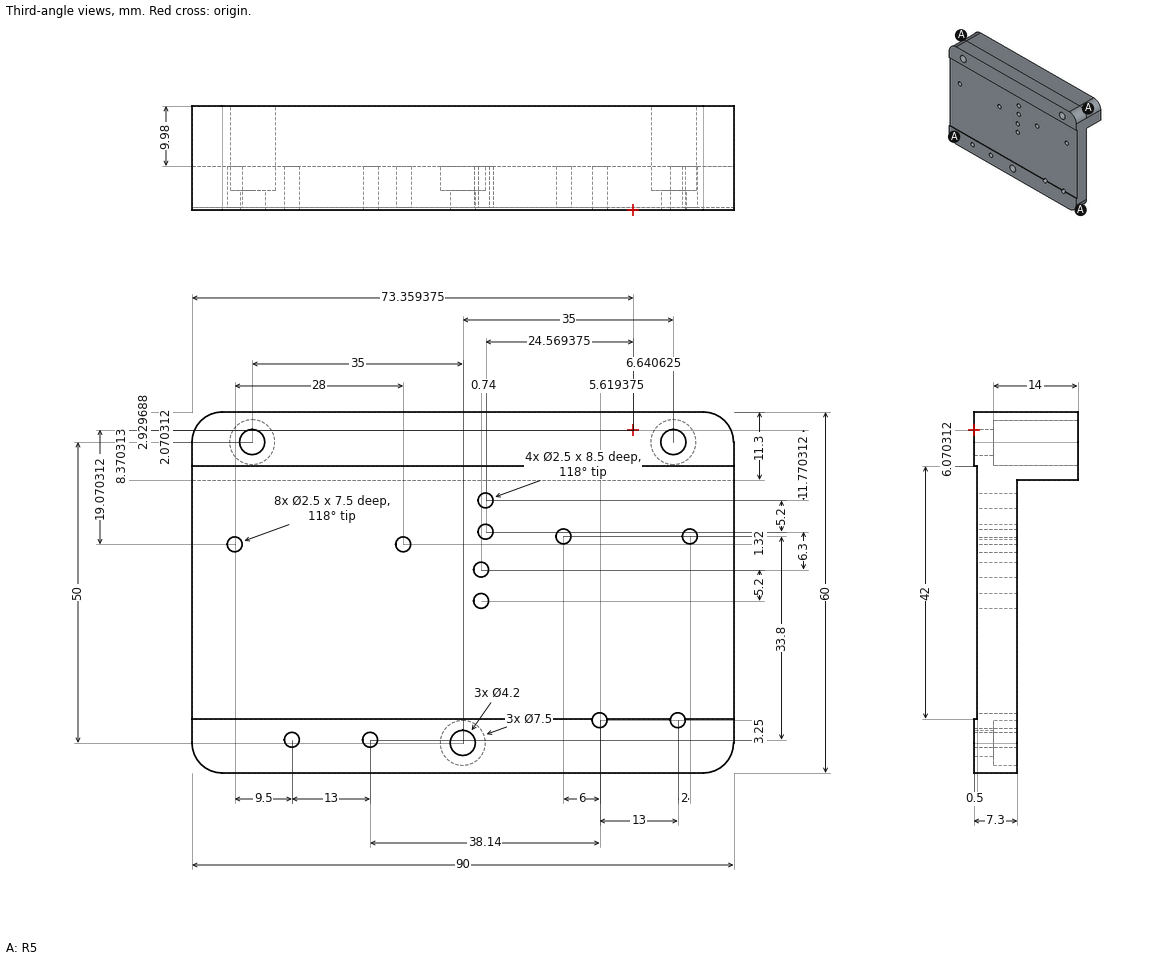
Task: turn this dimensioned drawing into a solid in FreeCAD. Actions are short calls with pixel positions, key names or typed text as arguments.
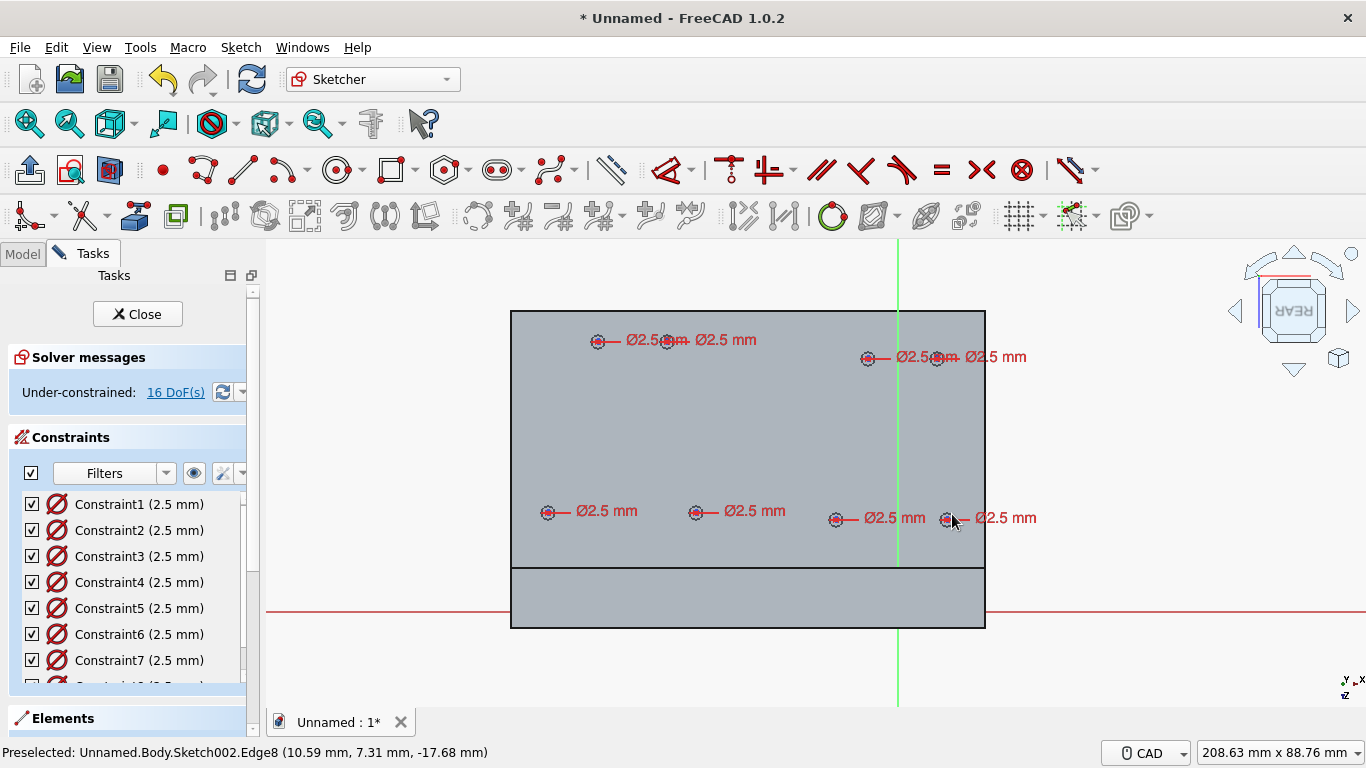
click(666, 170)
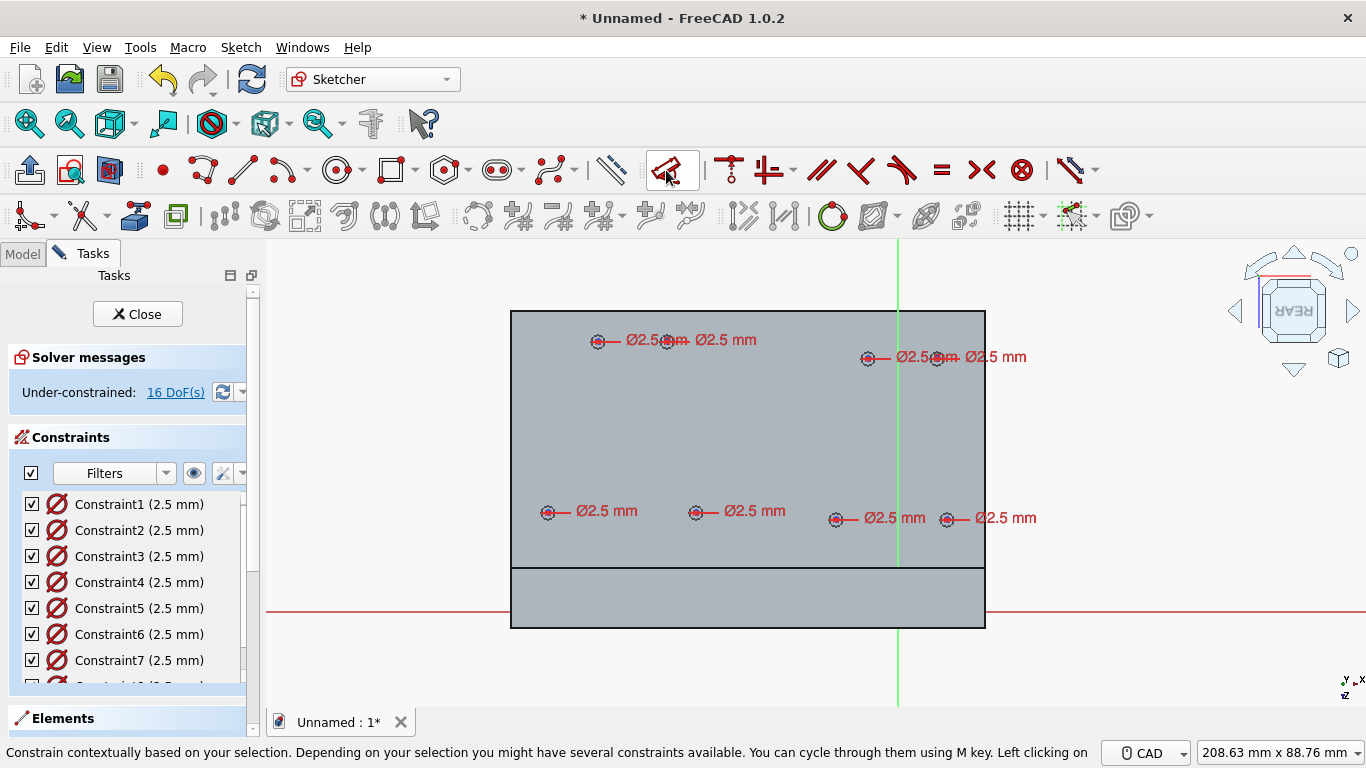
scroll(868, 359, up, 2)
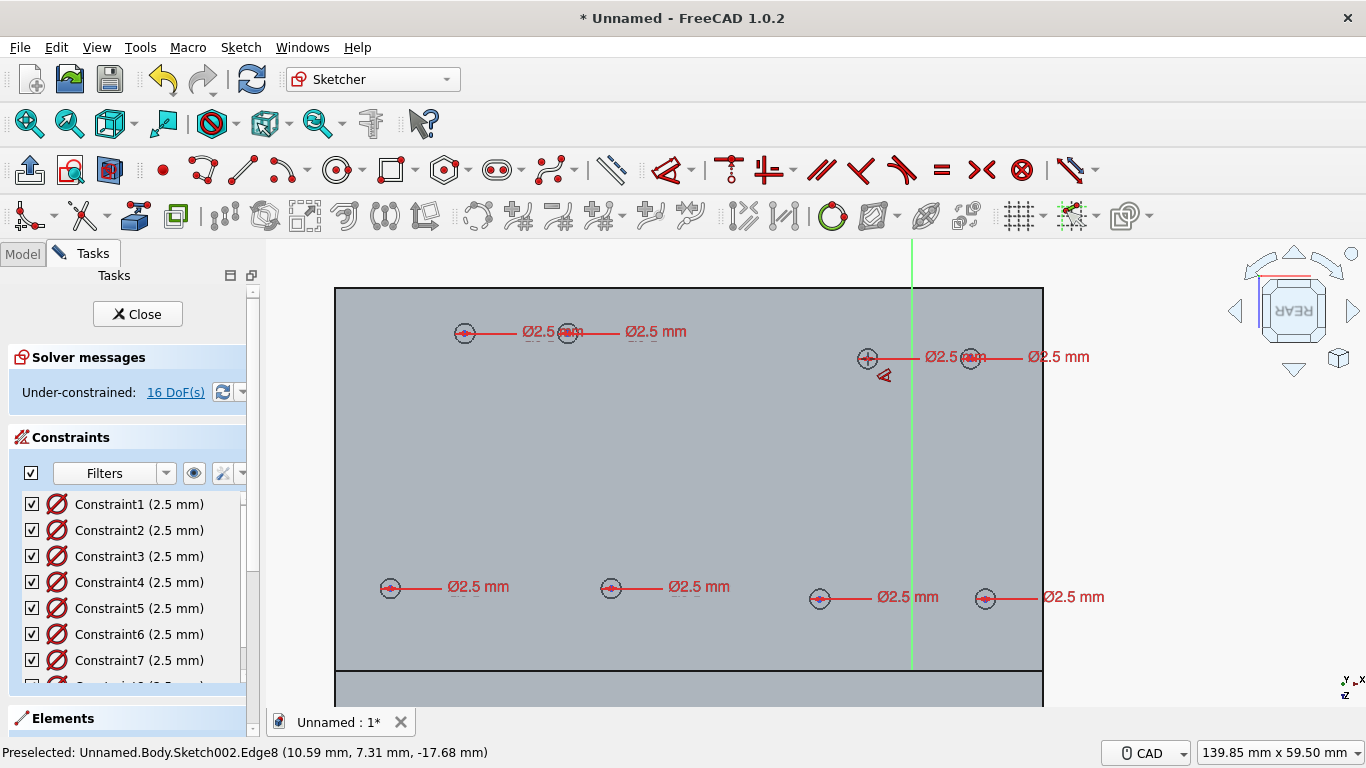
click(868, 359)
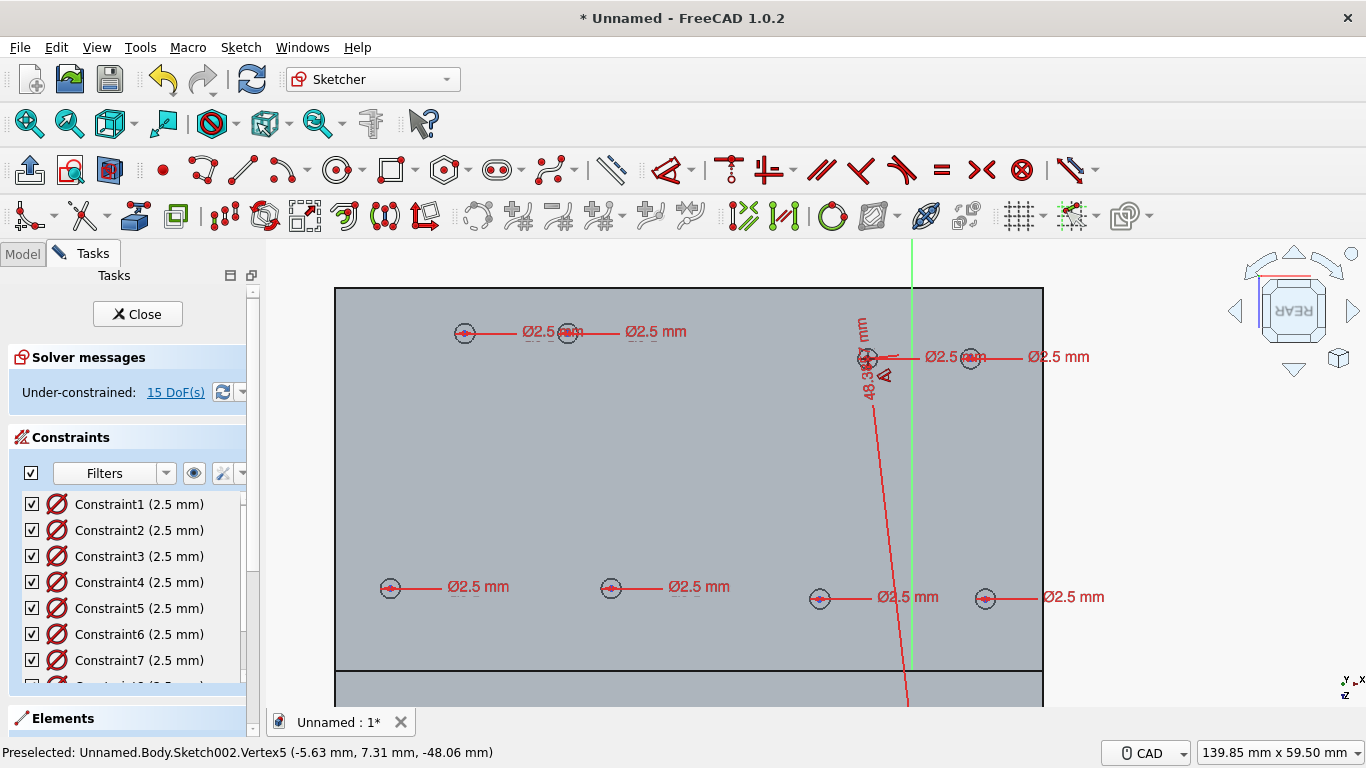
click(820, 599)
click(844, 325)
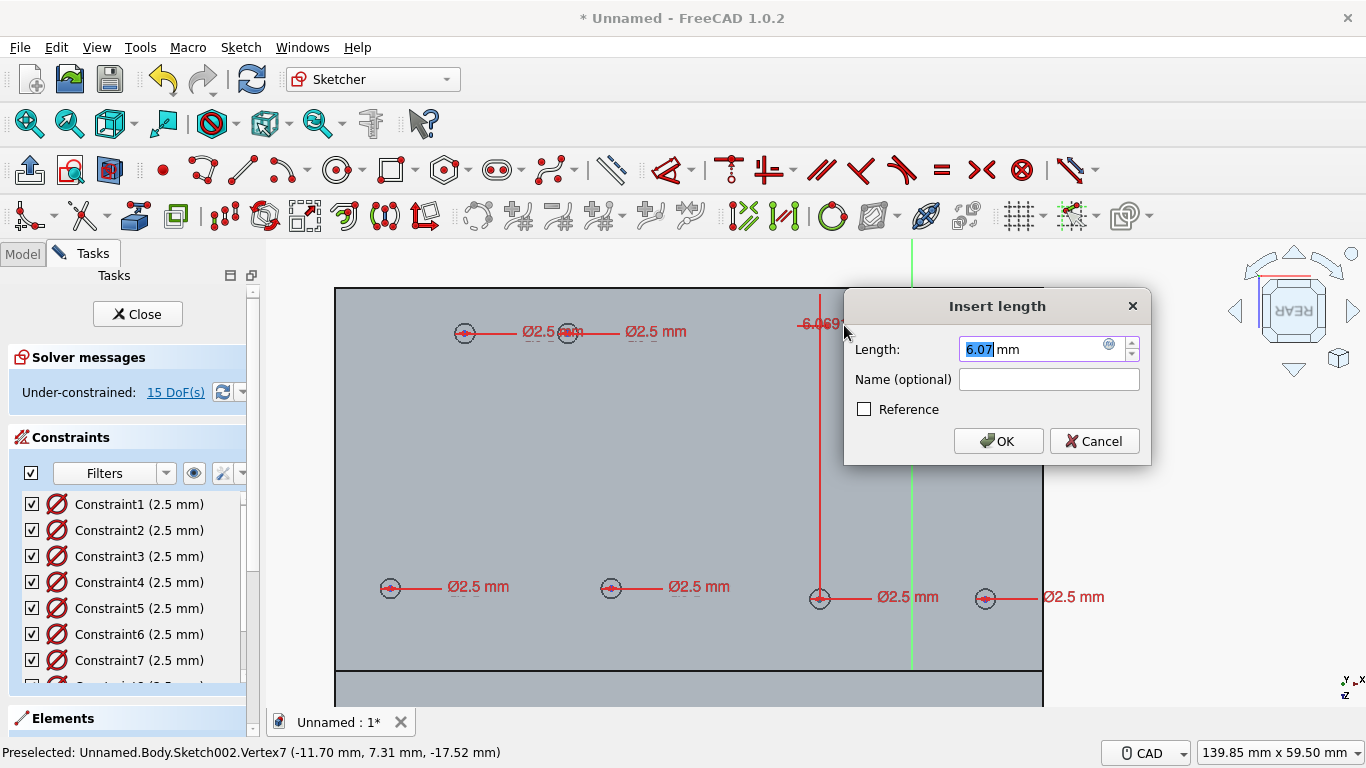
text(6)
key(Return)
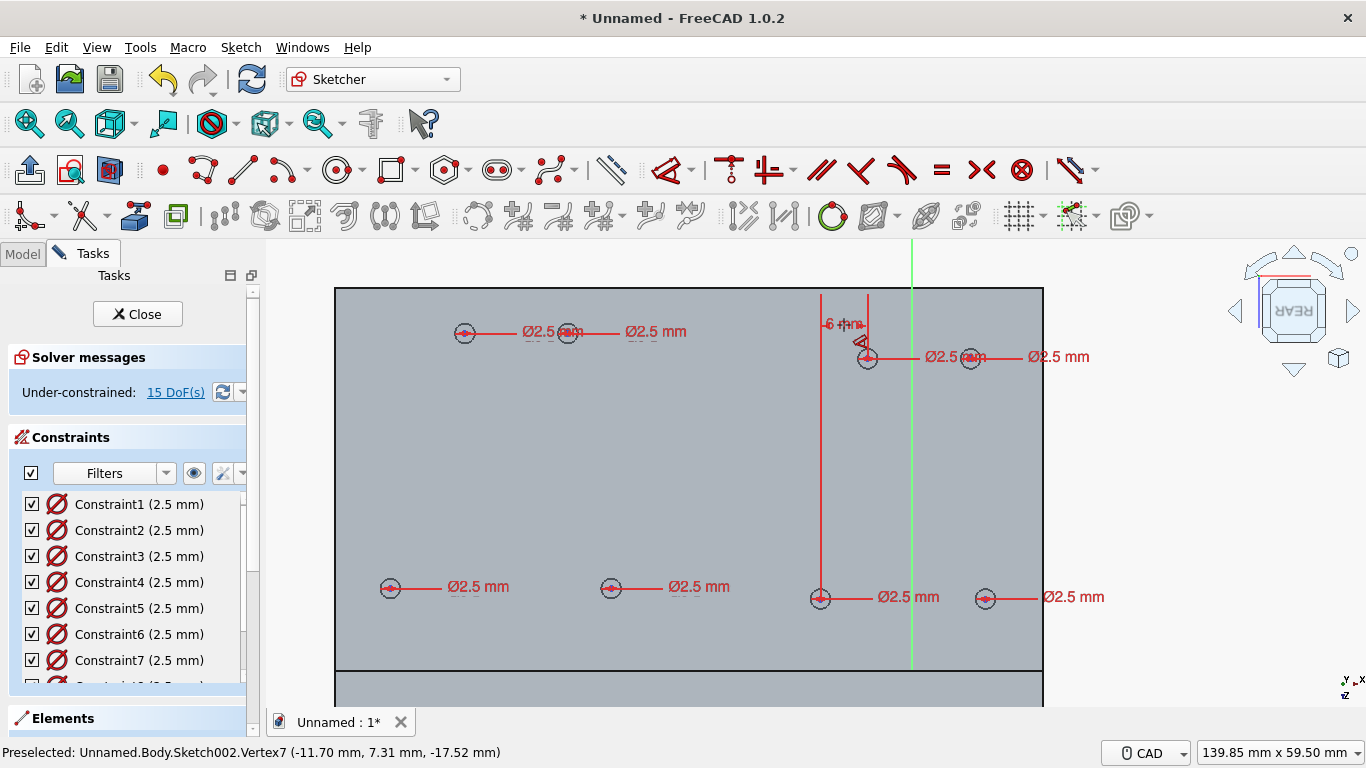
scroll(971, 359, up, 5)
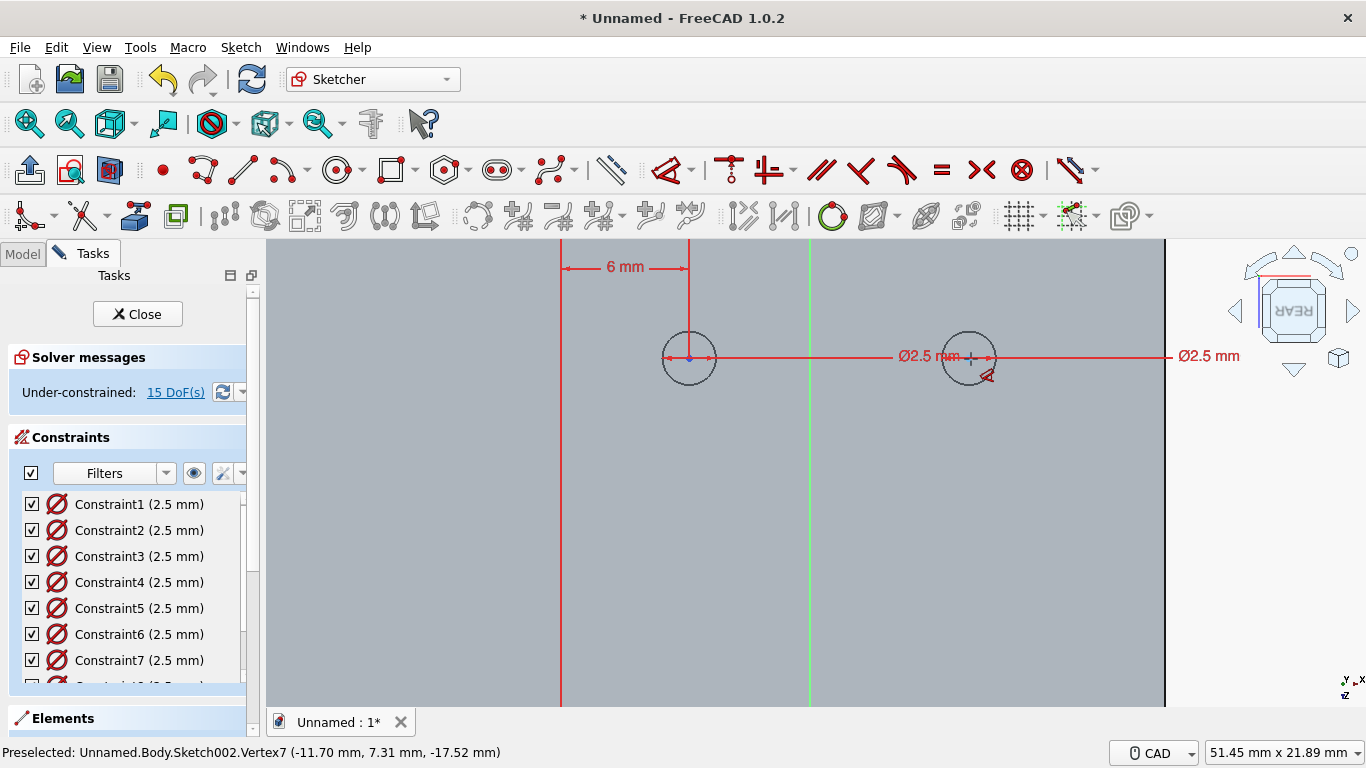
click(969, 358)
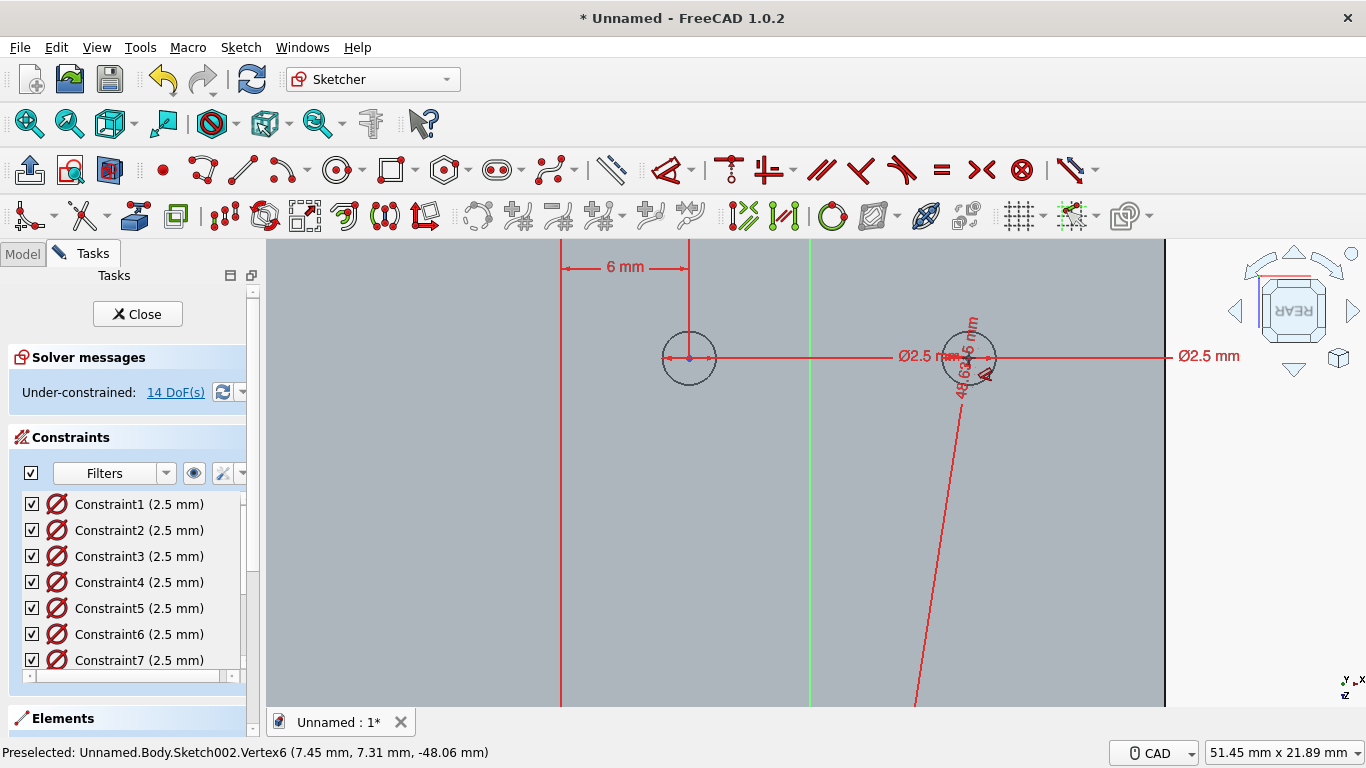
scroll(926, 359, down, 7)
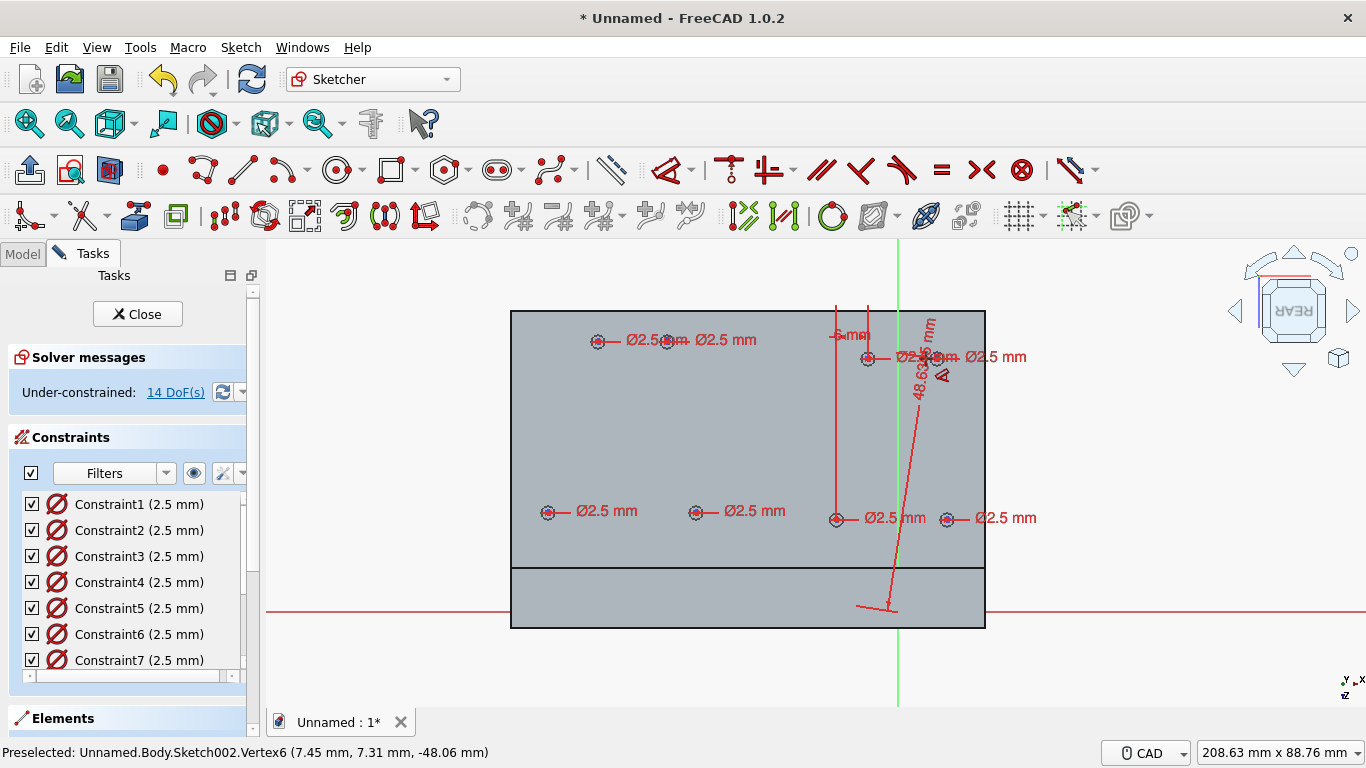
scroll(947, 520, up, 7)